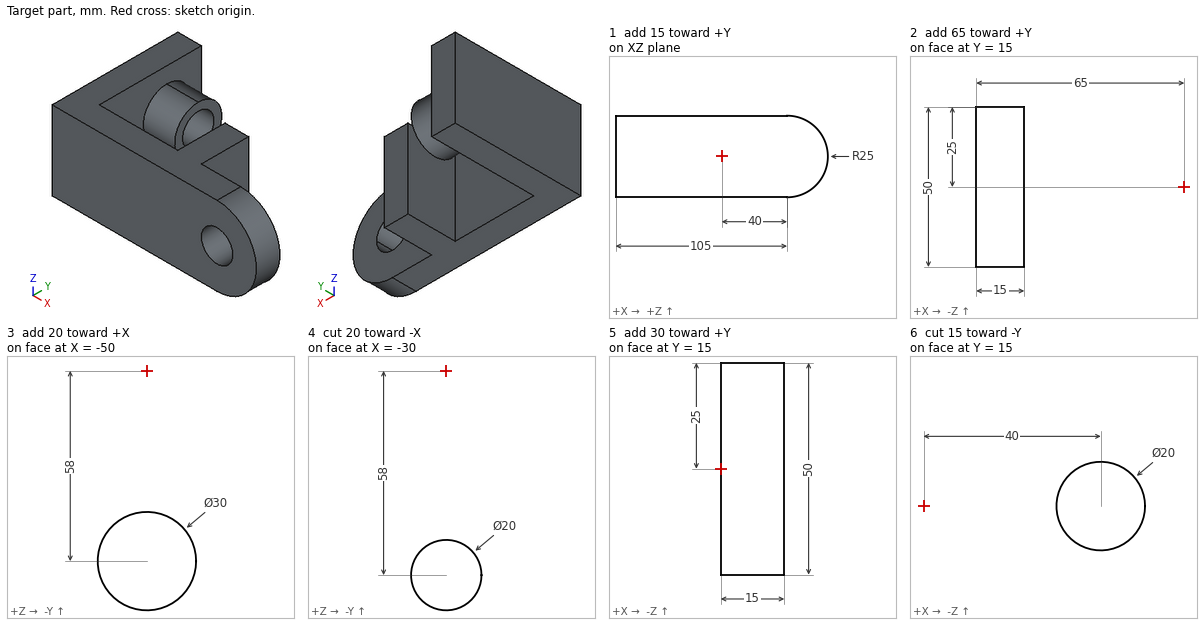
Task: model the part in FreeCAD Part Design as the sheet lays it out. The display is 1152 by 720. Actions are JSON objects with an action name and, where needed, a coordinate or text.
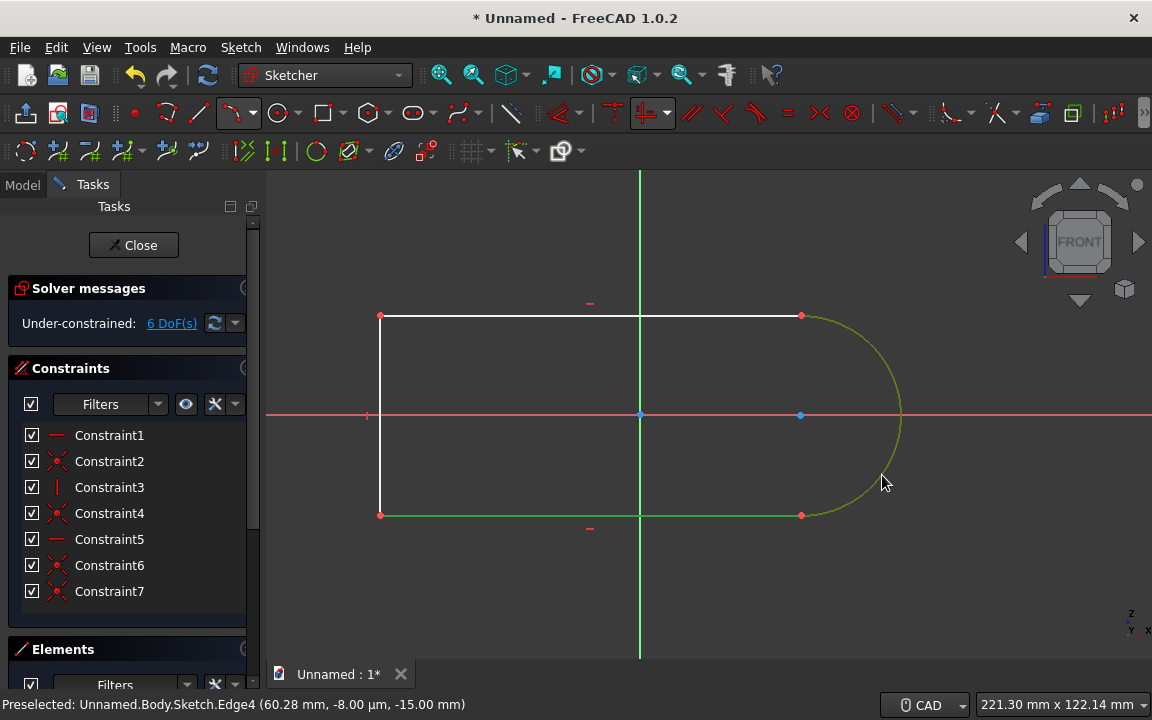
{"action": "left_click", "coordinate": [756, 114]}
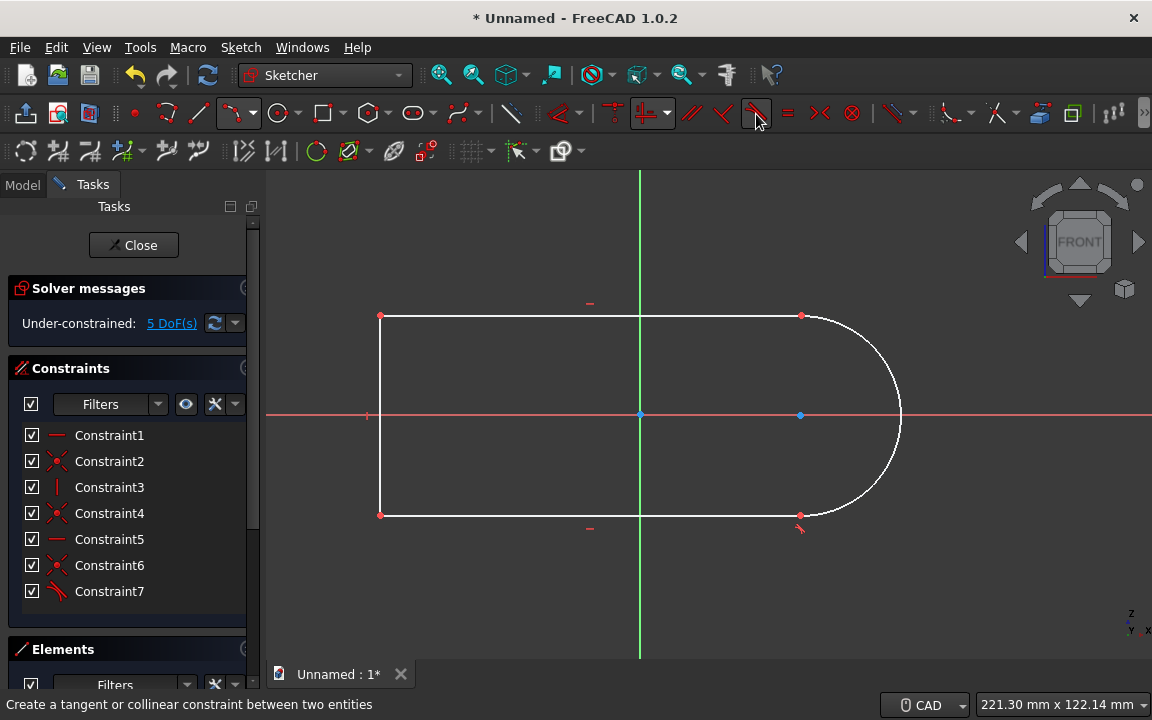
{"action": "left_click", "coordinate": [506, 316]}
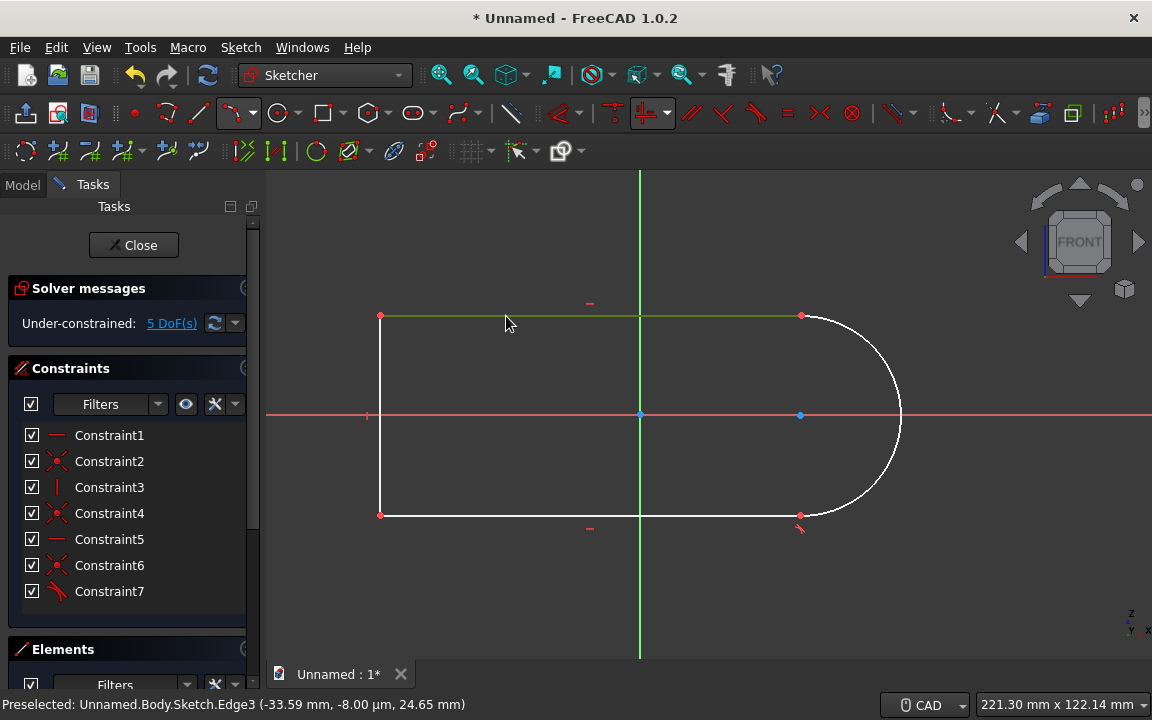
{"action": "left_click", "coordinate": [882, 475]}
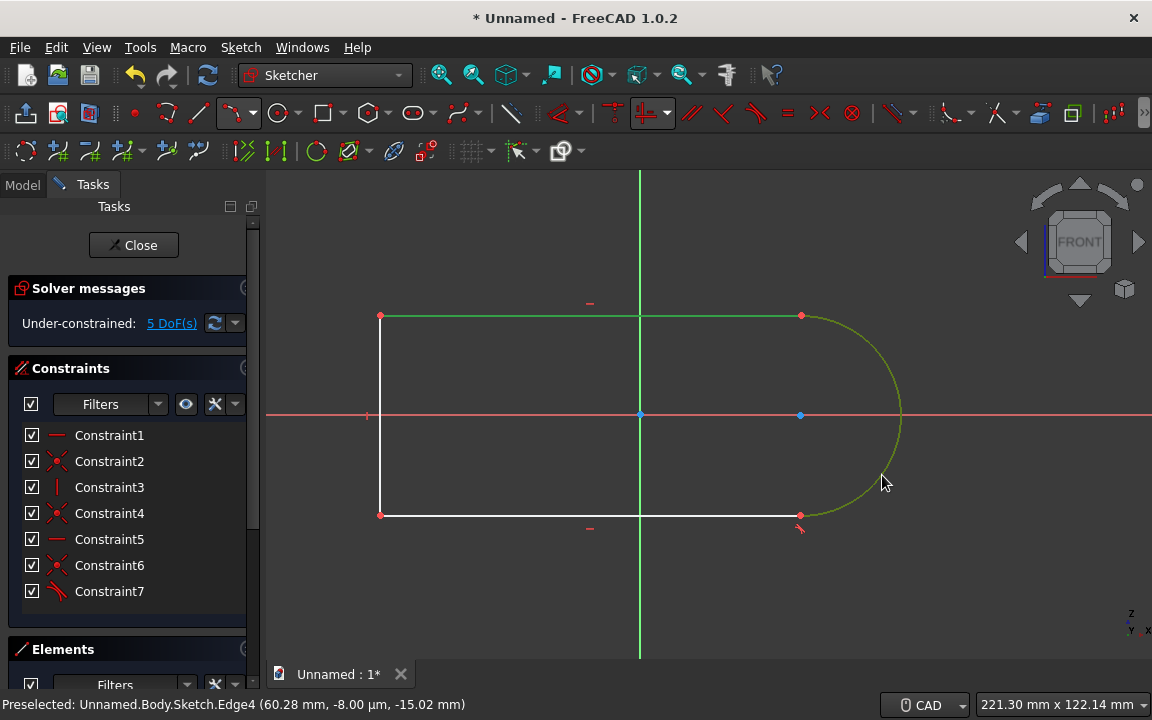
{"action": "left_click", "coordinate": [756, 114]}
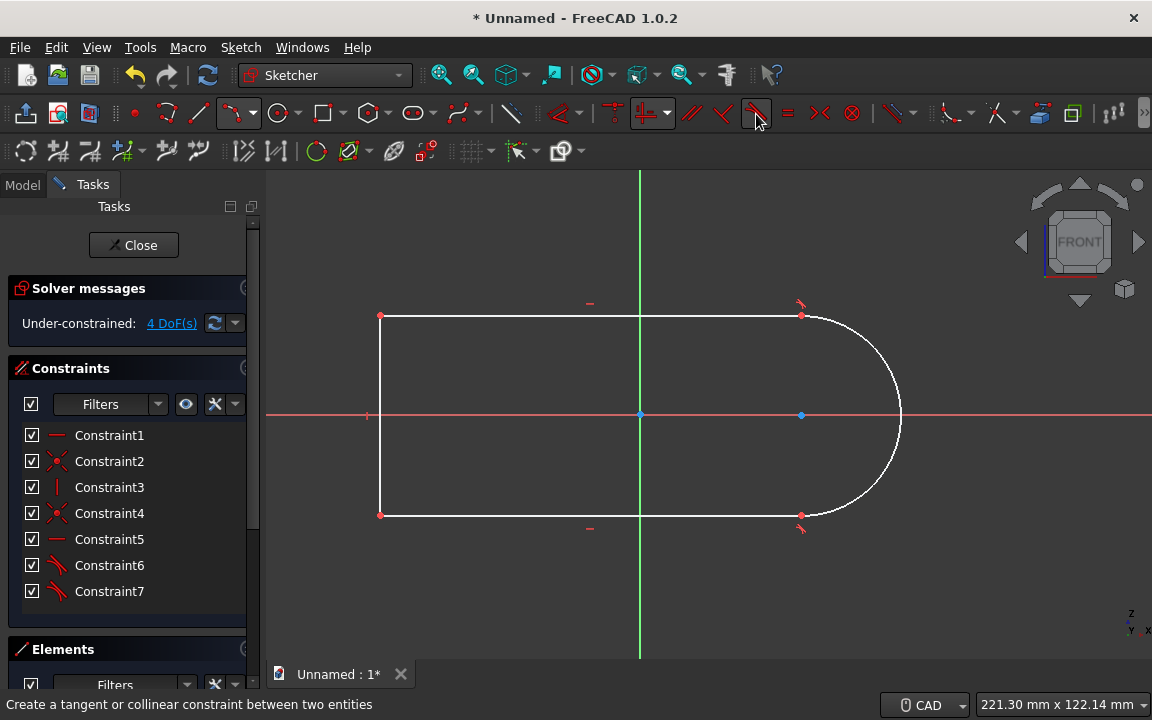
{"action": "left_click", "coordinate": [801, 416]}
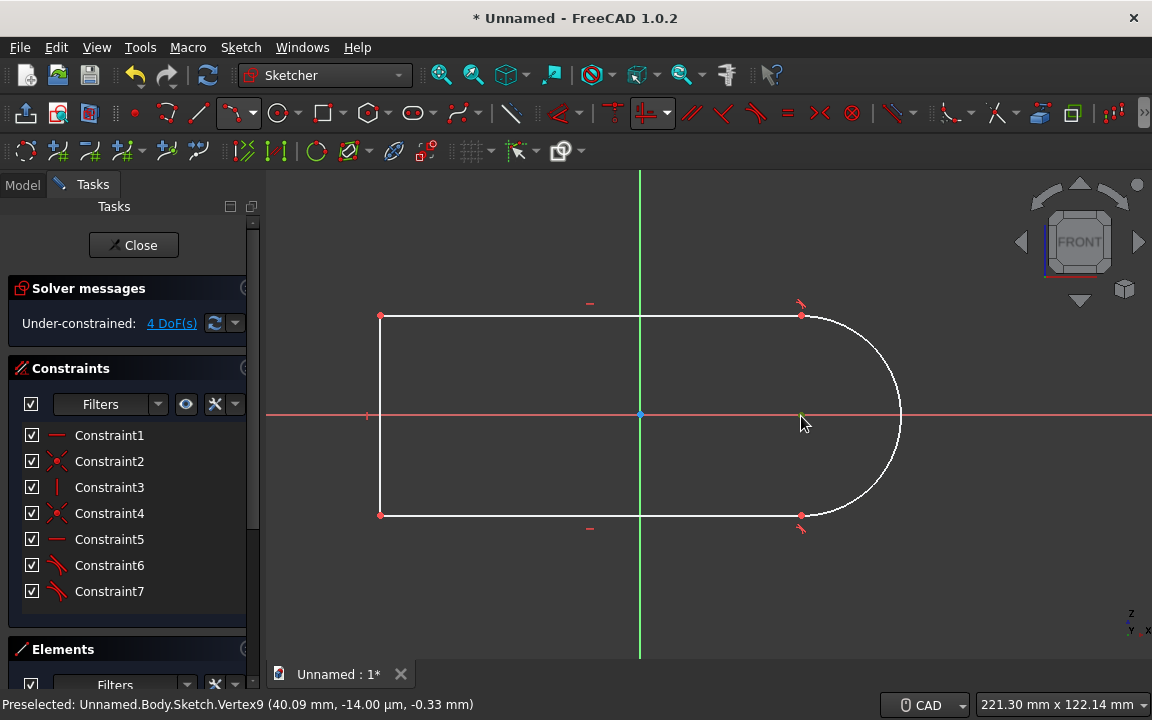
{"action": "left_click", "coordinate": [344, 415]}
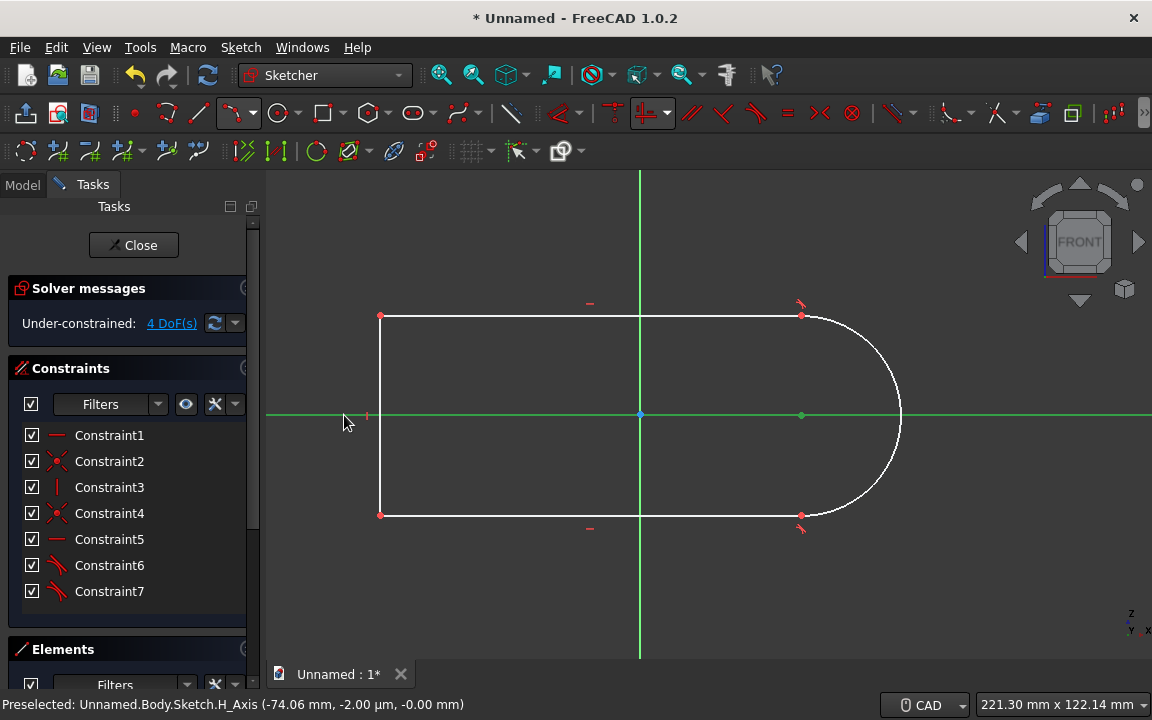
{"action": "left_click", "coordinate": [614, 114]}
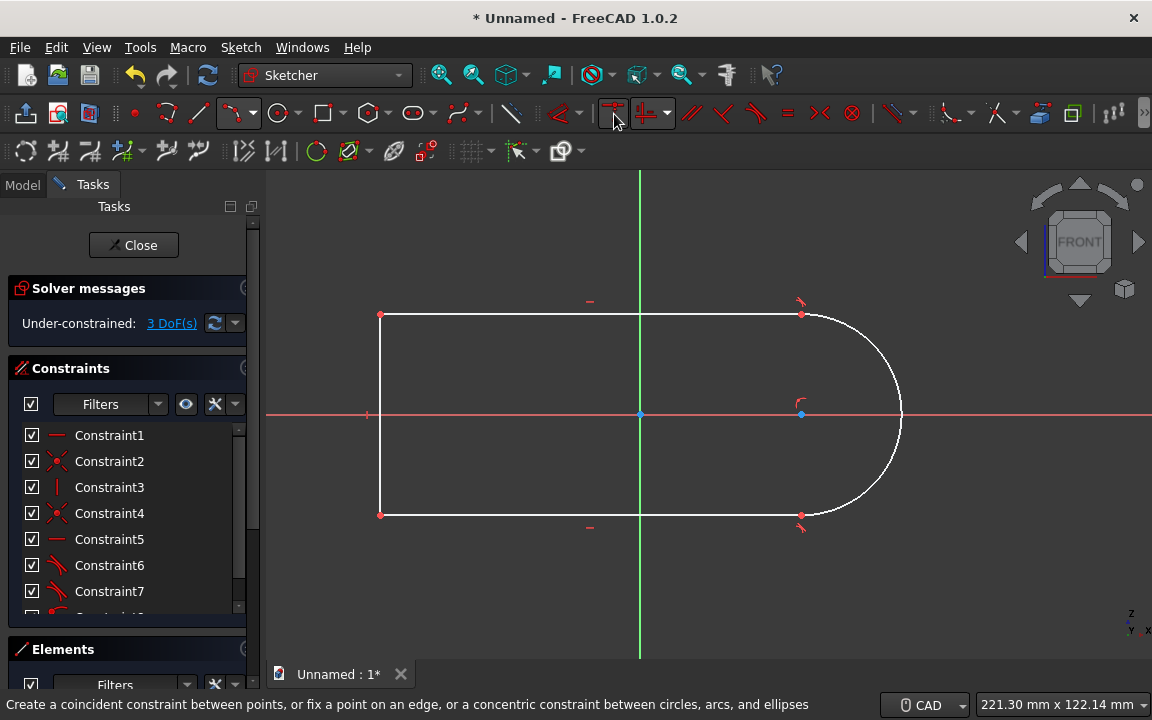
{"action": "left_click", "coordinate": [558, 114]}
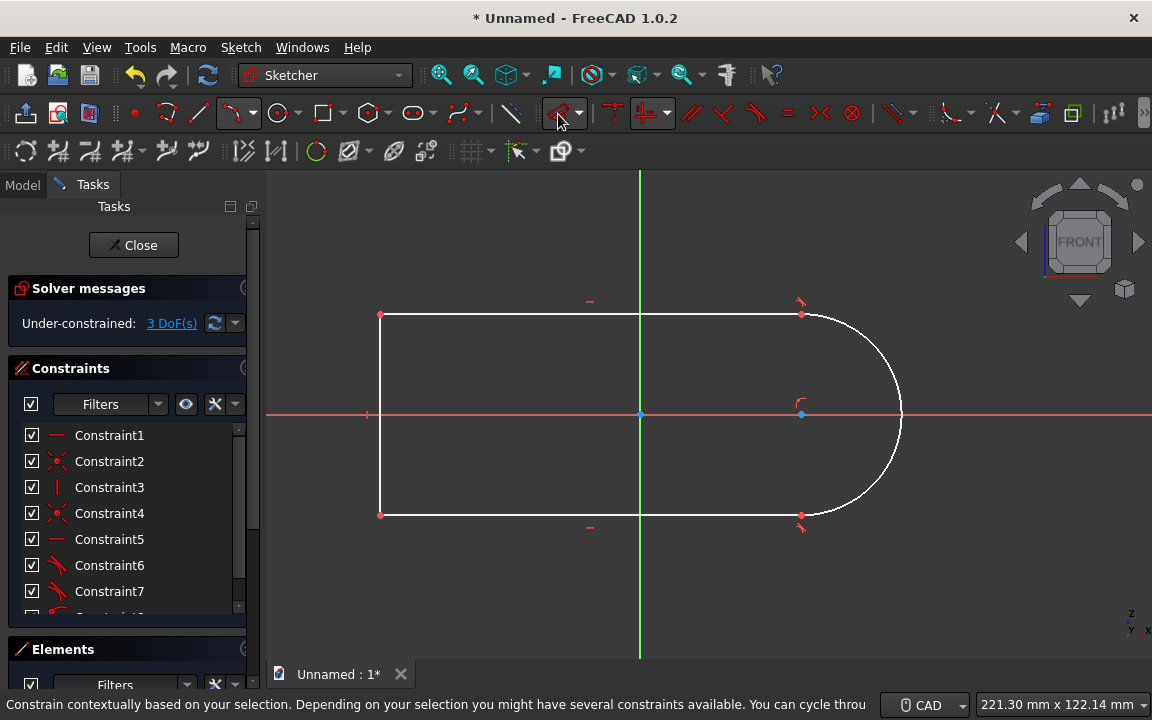
{"action": "left_click", "coordinate": [882, 474]}
{"action": "left_click", "coordinate": [908, 493]}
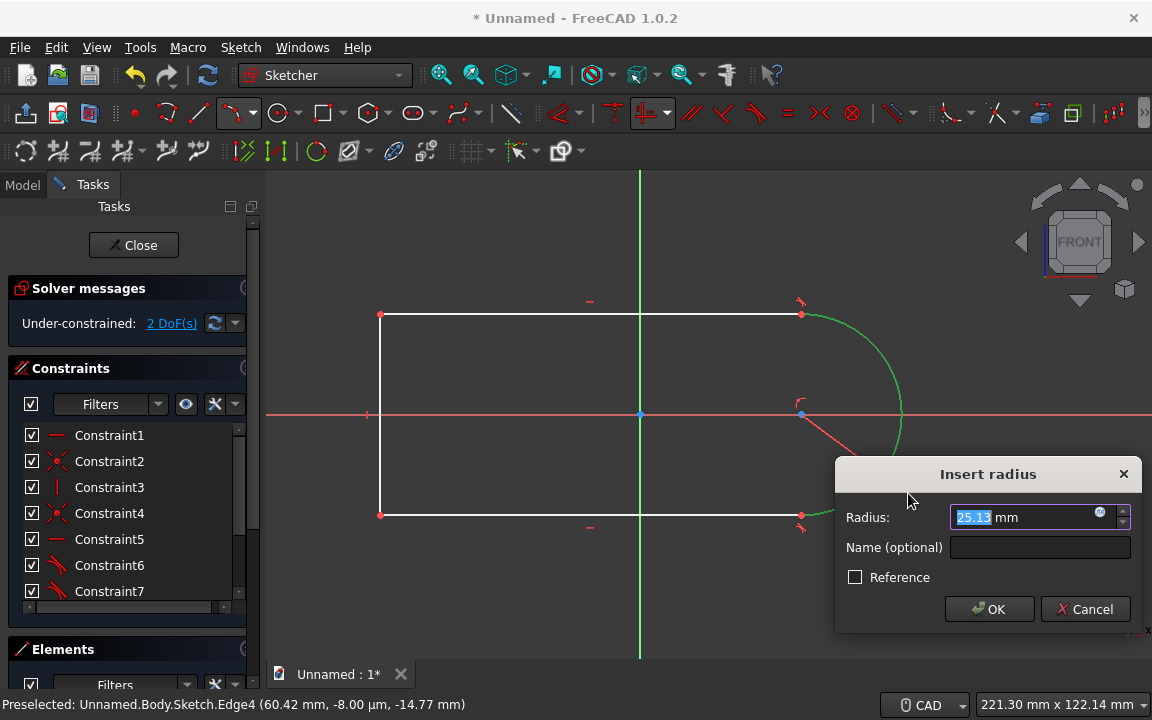
{"action": "type", "text": "25"}
{"action": "key", "text": "Return"}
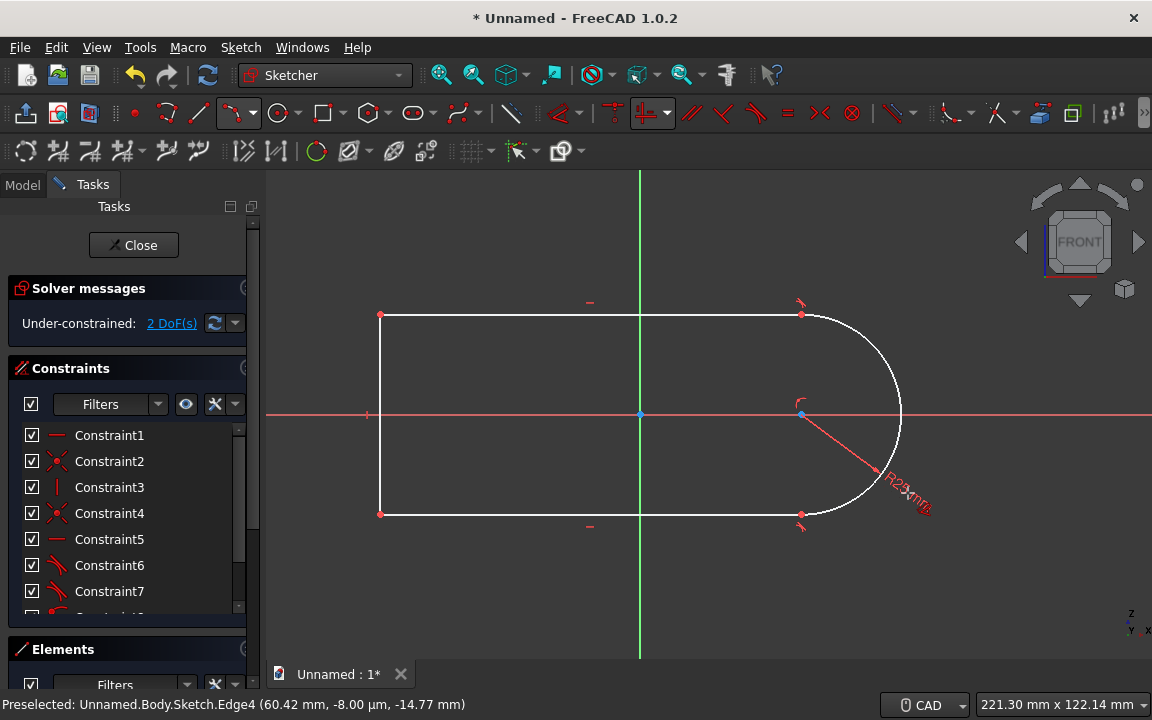
{"action": "left_click", "coordinate": [675, 515]}
{"action": "left_click", "coordinate": [591, 549]}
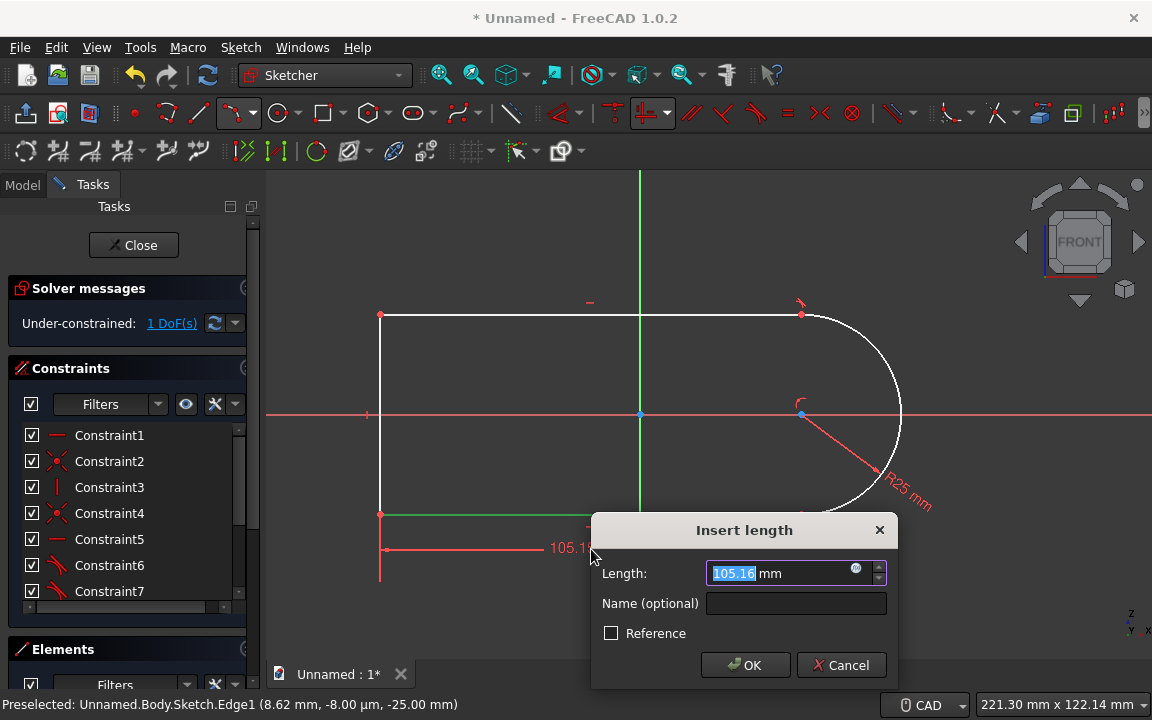
{"action": "type", "text": "105"}
{"action": "key", "text": "Return"}